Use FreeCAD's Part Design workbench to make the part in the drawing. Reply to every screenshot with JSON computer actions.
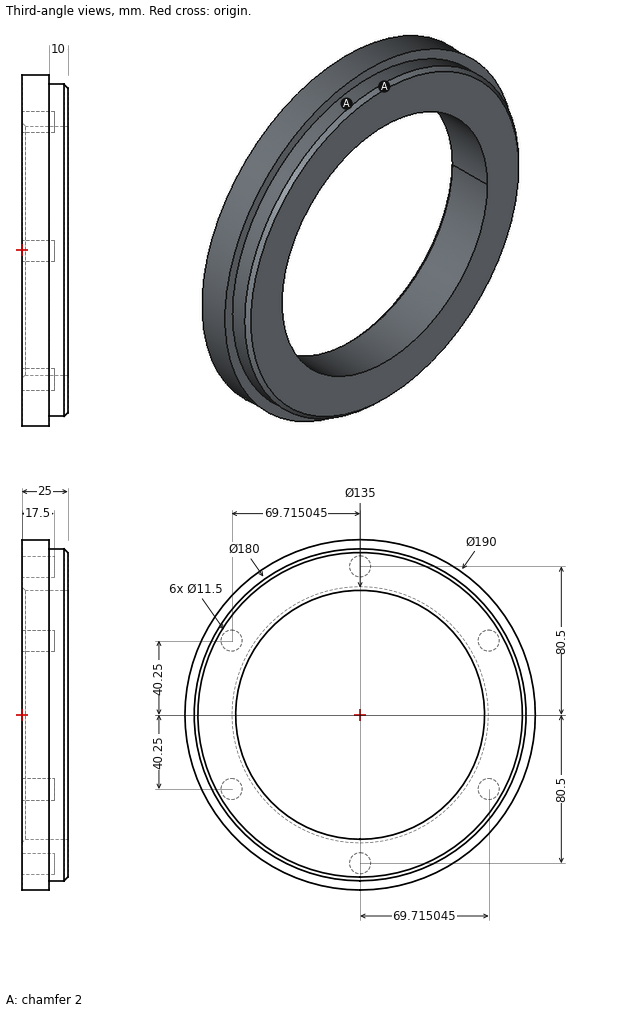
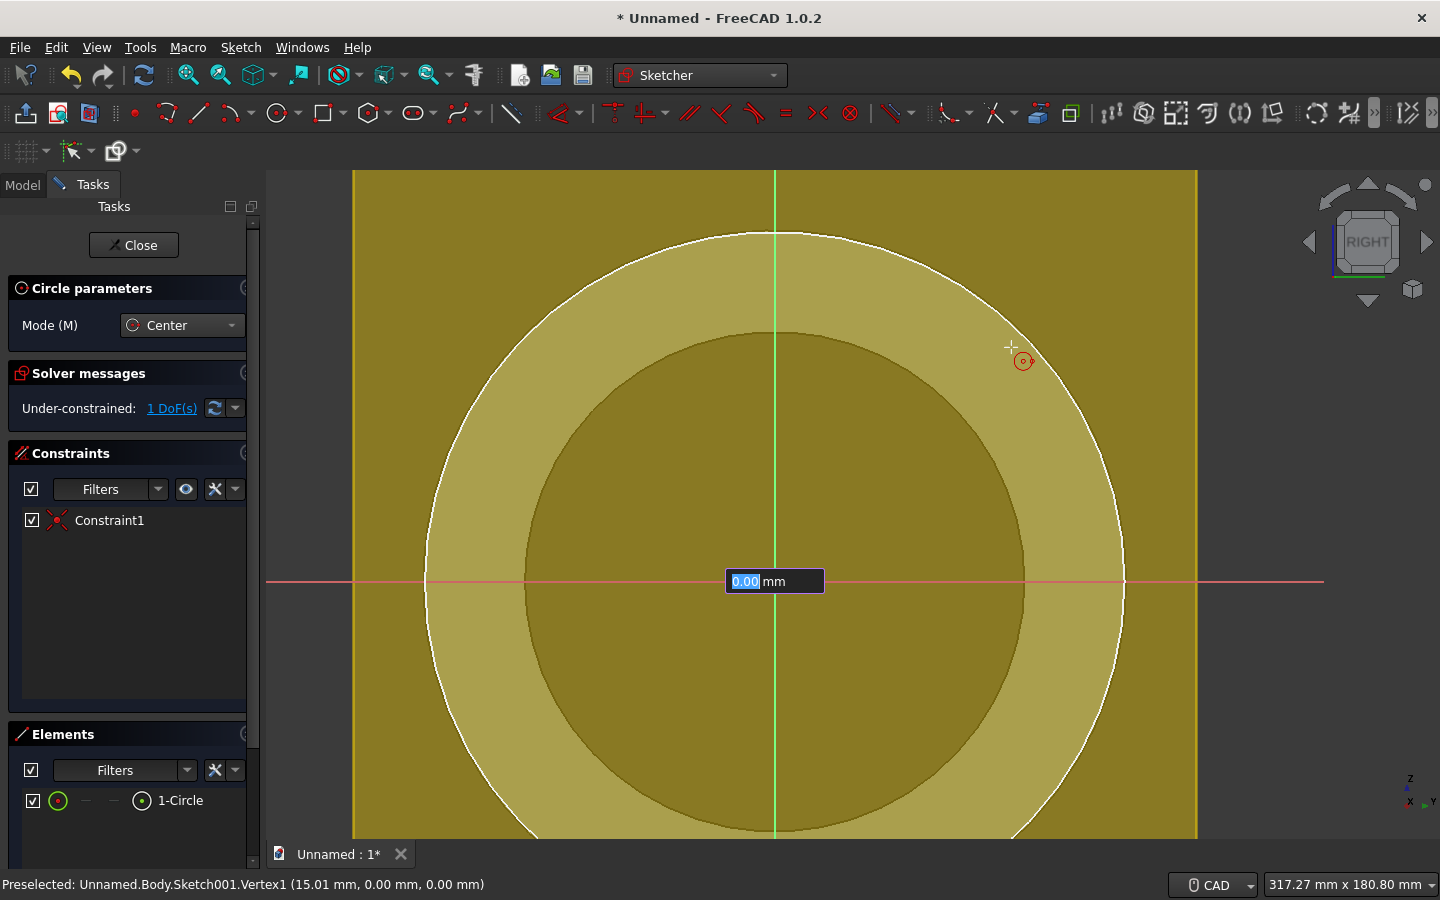
{"action": "left_click", "coordinate": [1010, 346]}
{"action": "key", "text": "Escape"}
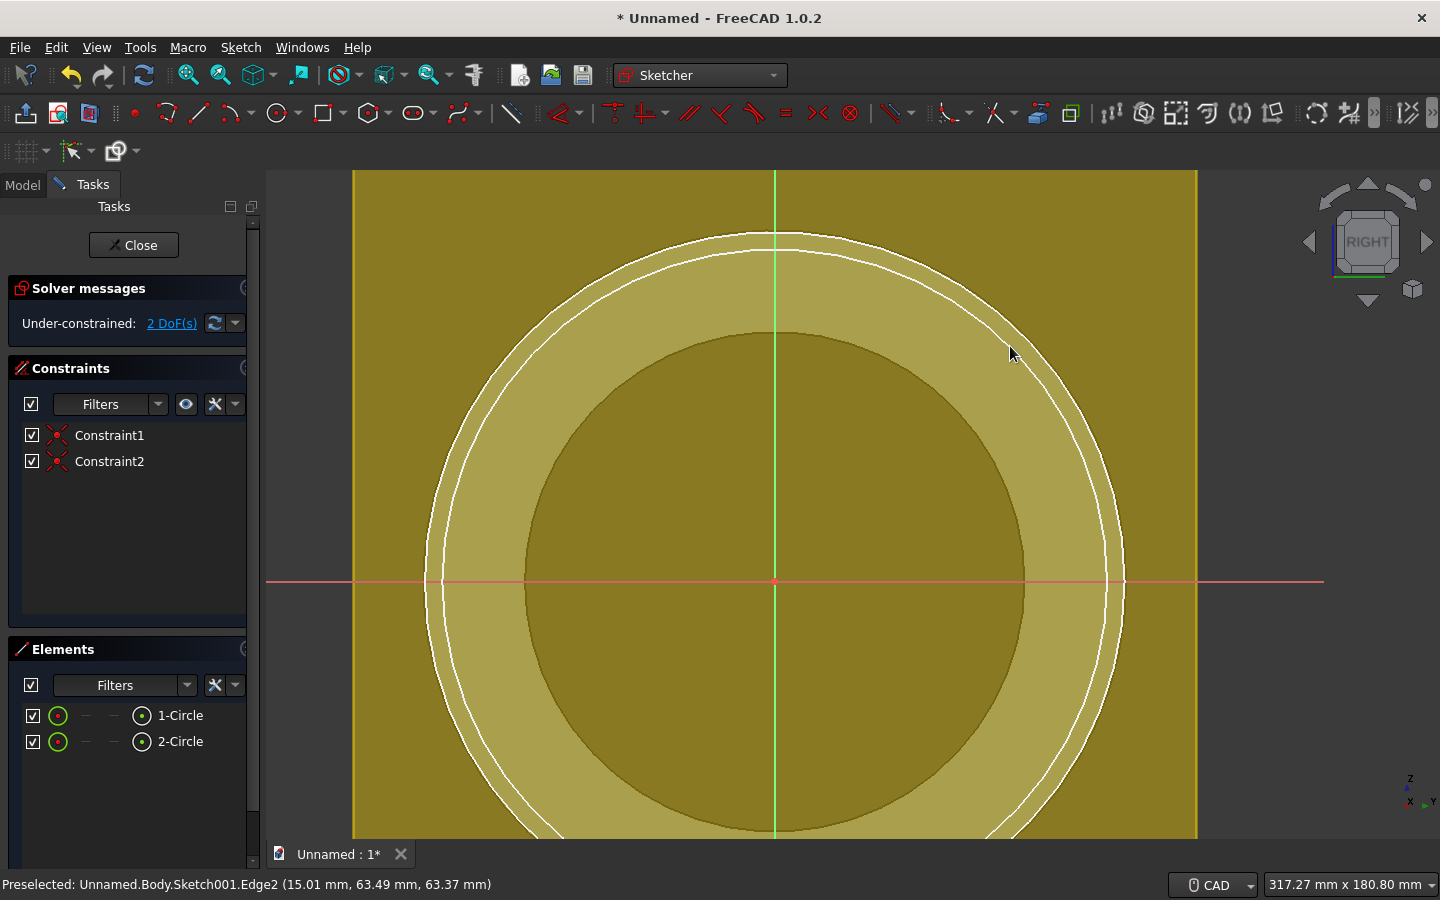
{"action": "left_click", "coordinate": [558, 114]}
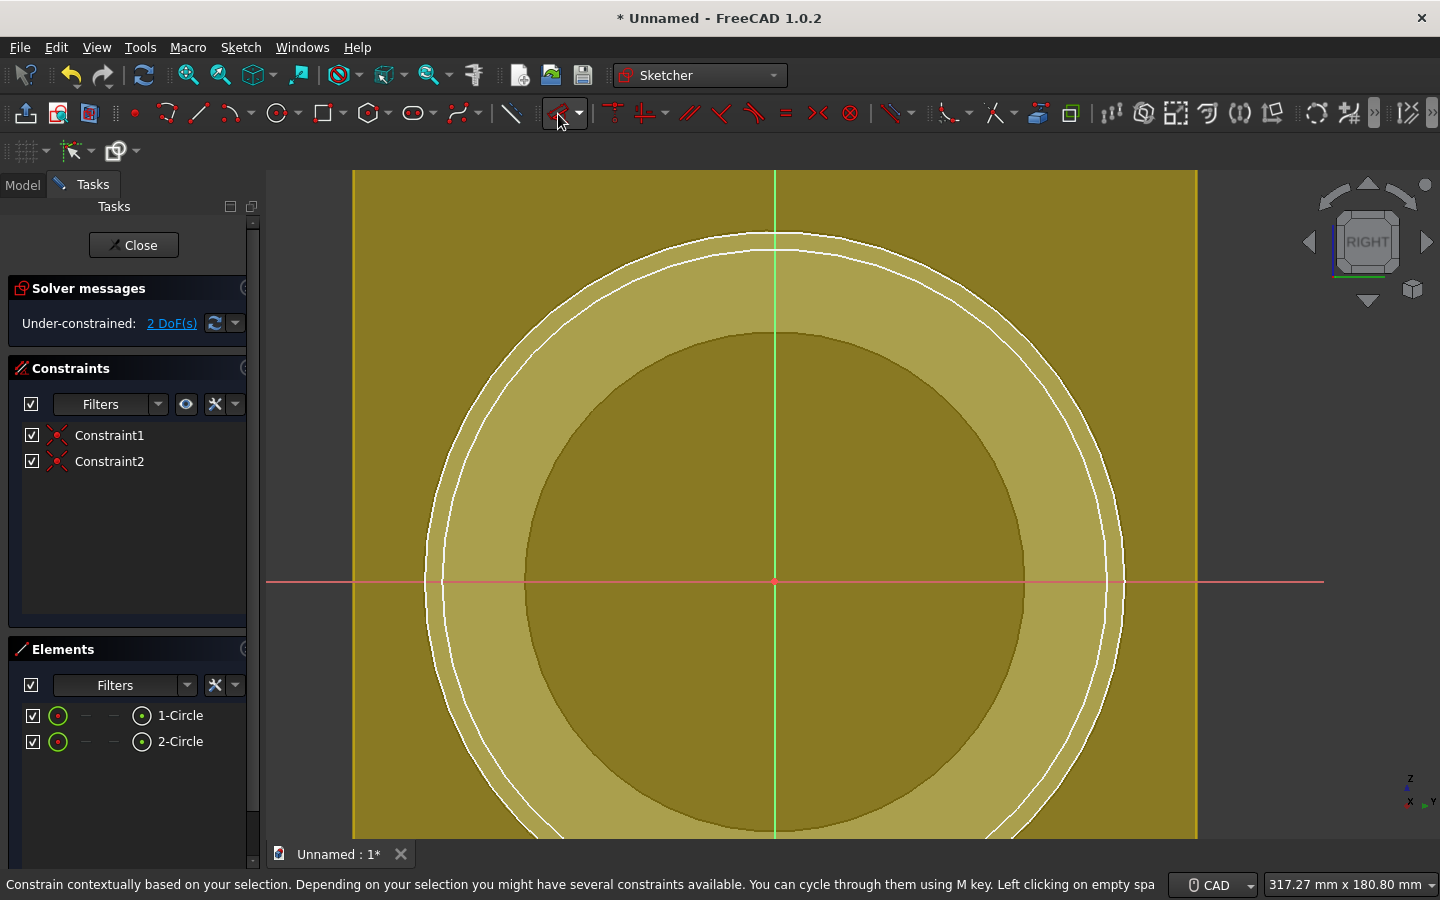
{"action": "left_click", "coordinate": [1021, 334]}
{"action": "left_click", "coordinate": [1044, 311]}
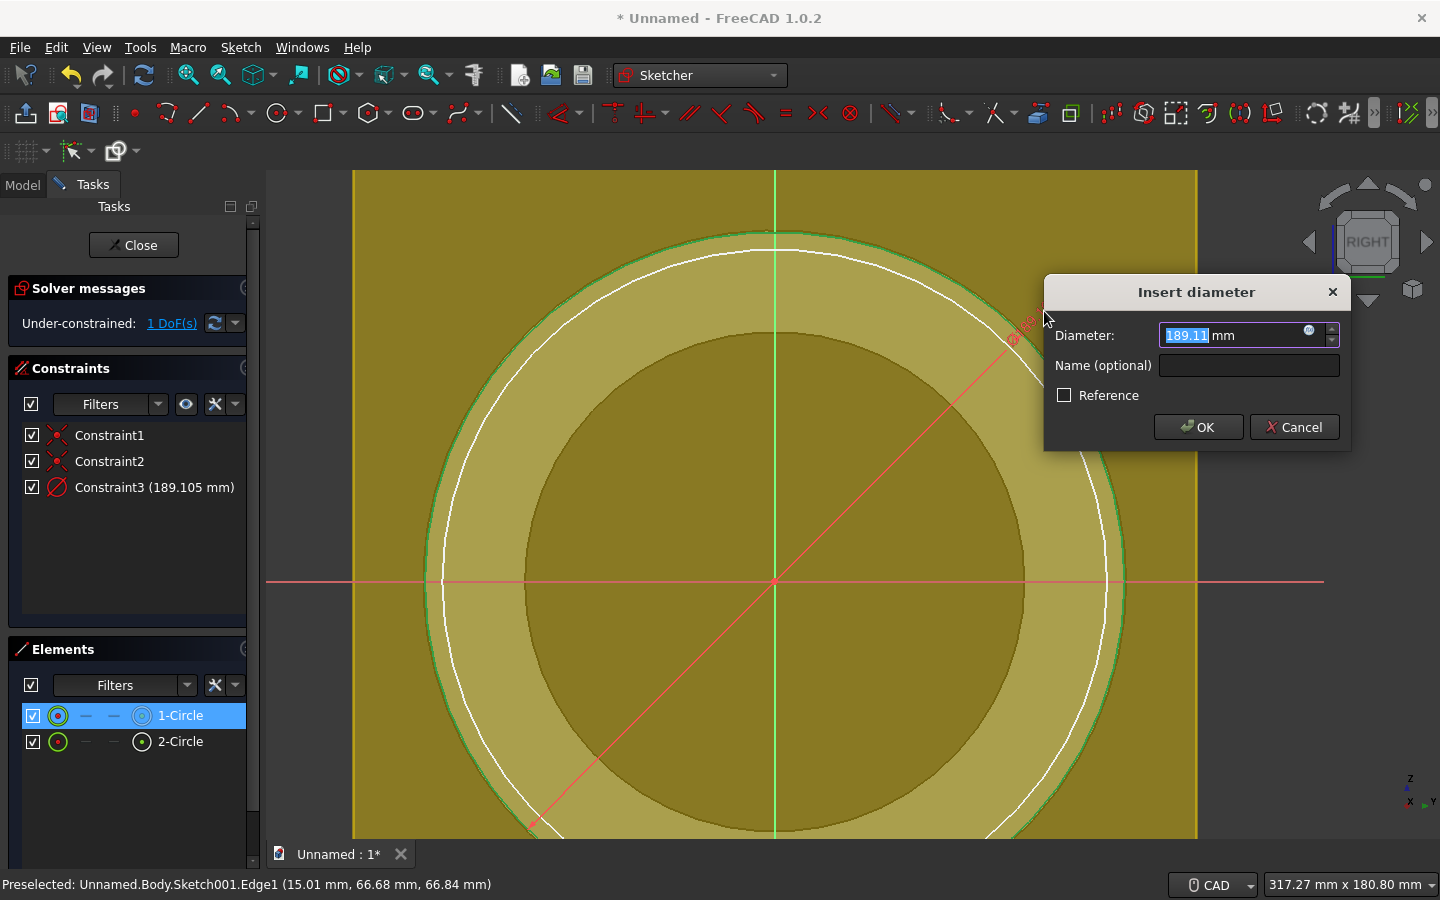
{"action": "type", "text": "190"}
{"action": "key", "text": "Return"}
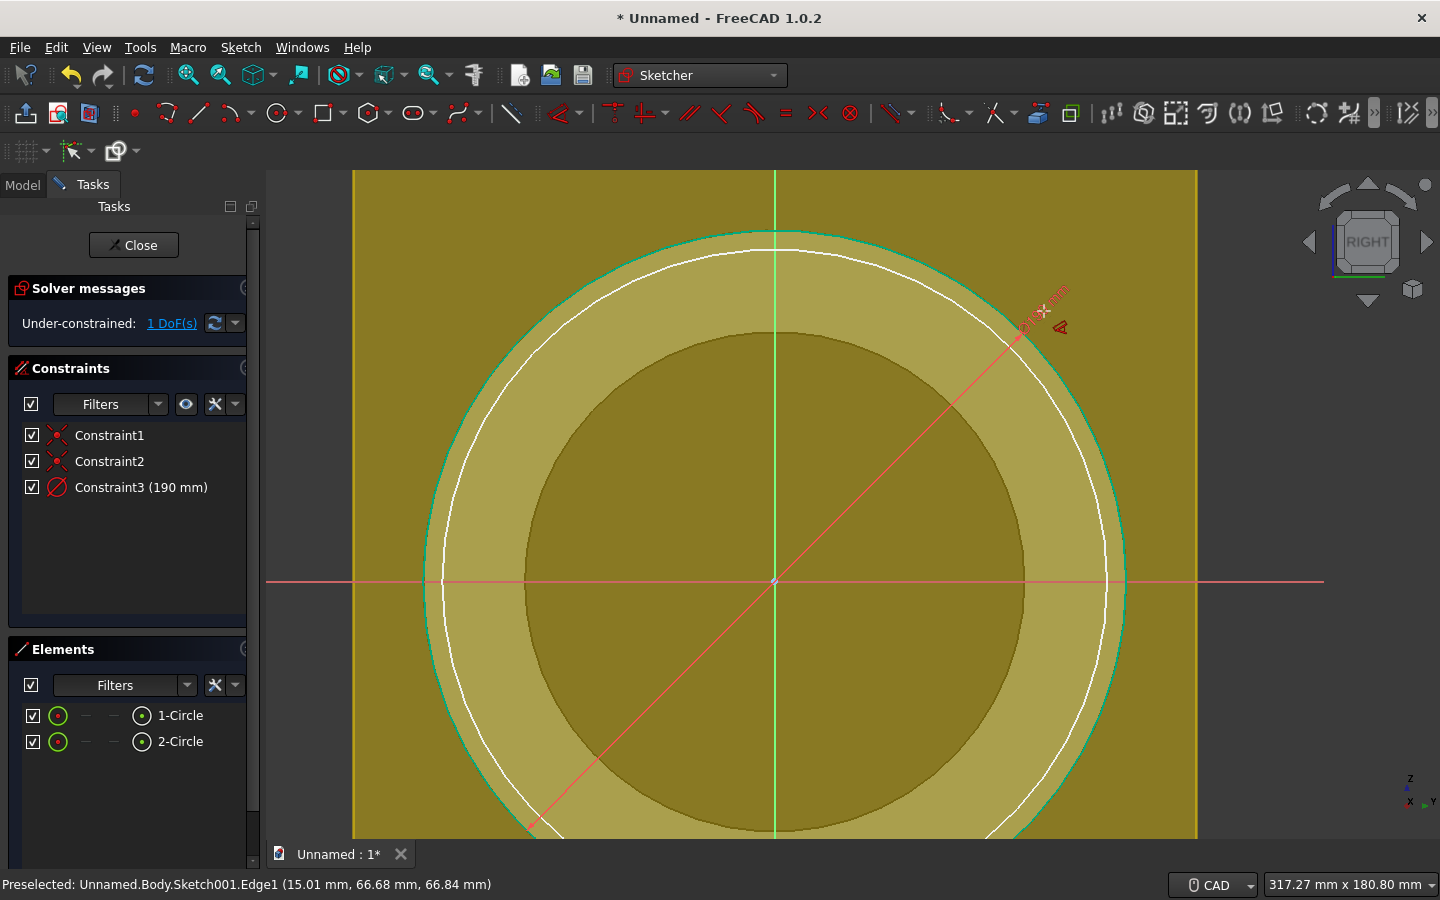
{"action": "left_click", "coordinate": [1009, 346]}
{"action": "left_click", "coordinate": [1146, 472]}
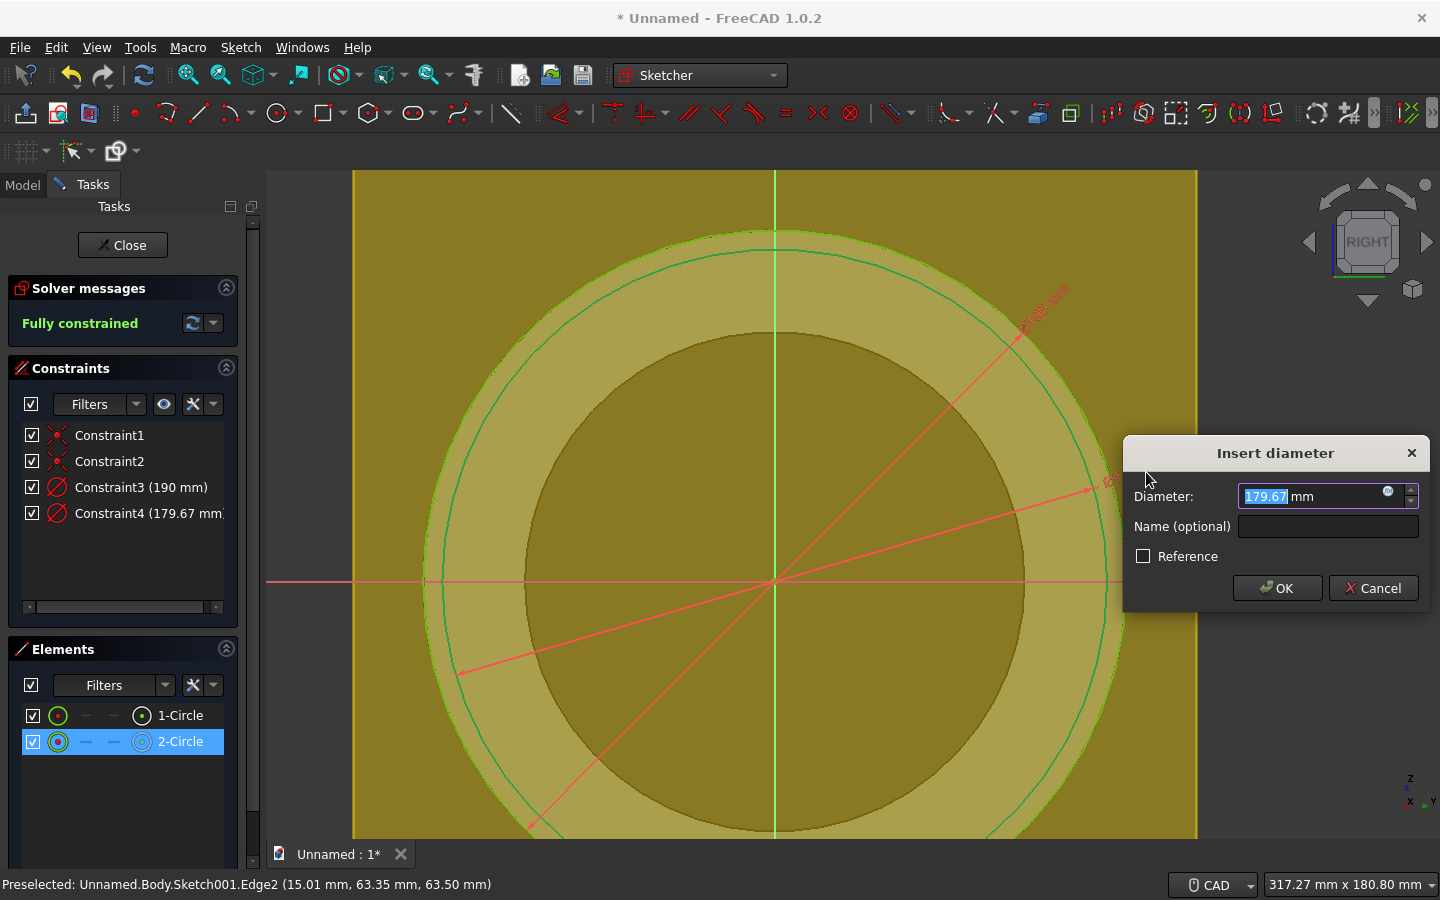
{"action": "type", "text": "180"}
{"action": "key", "text": "Return"}
{"action": "key", "text": "Escape"}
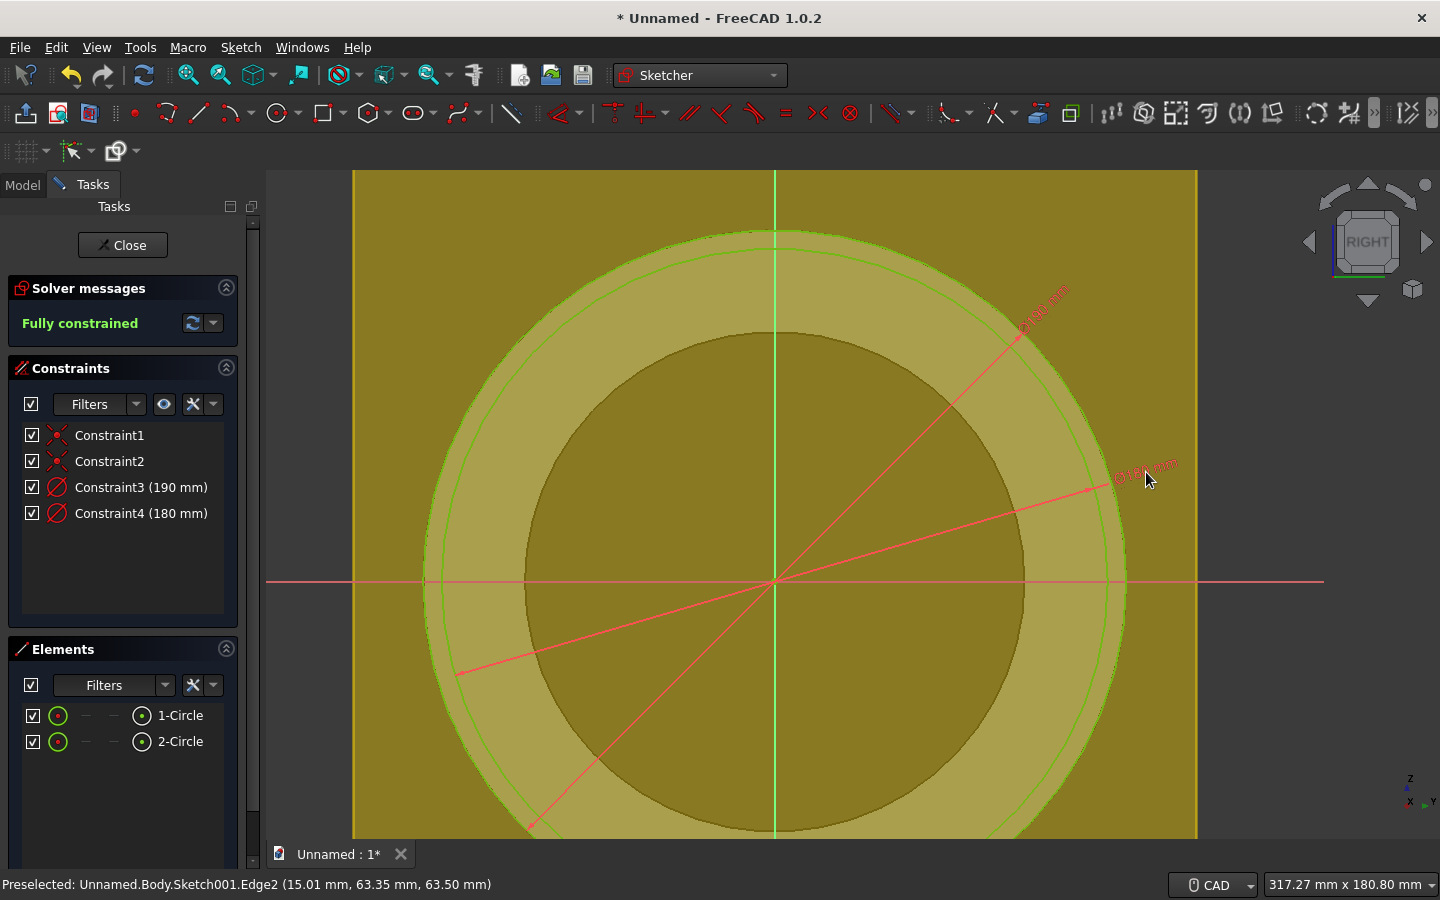
{"action": "left_click", "coordinate": [123, 245]}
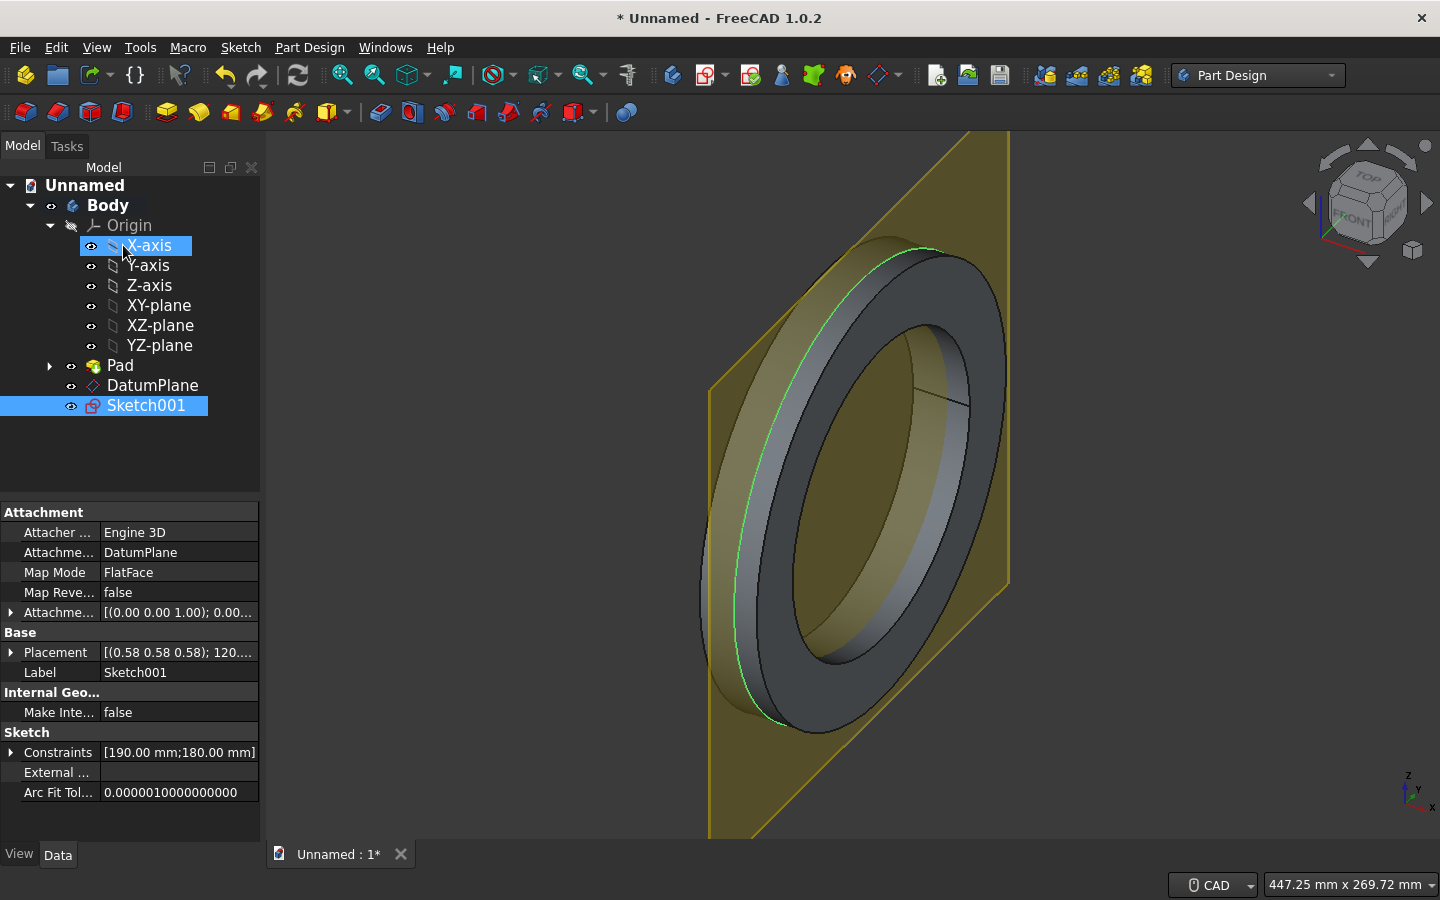
{"action": "left_click", "coordinate": [382, 112]}